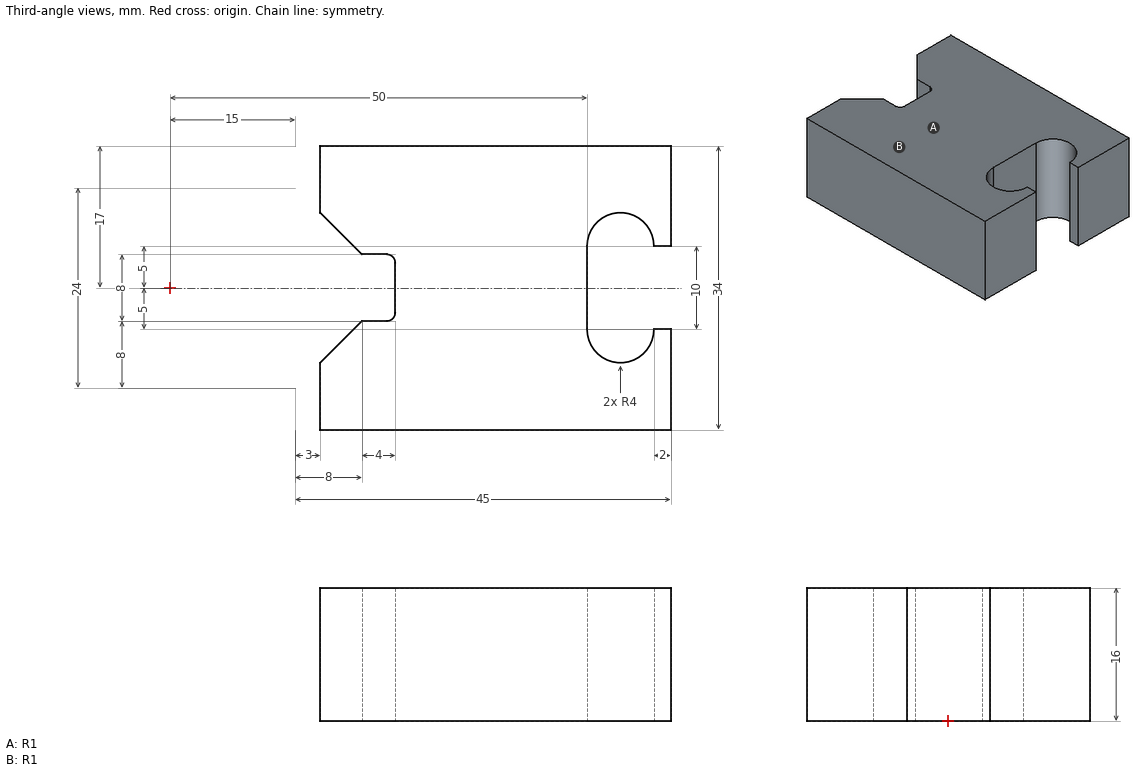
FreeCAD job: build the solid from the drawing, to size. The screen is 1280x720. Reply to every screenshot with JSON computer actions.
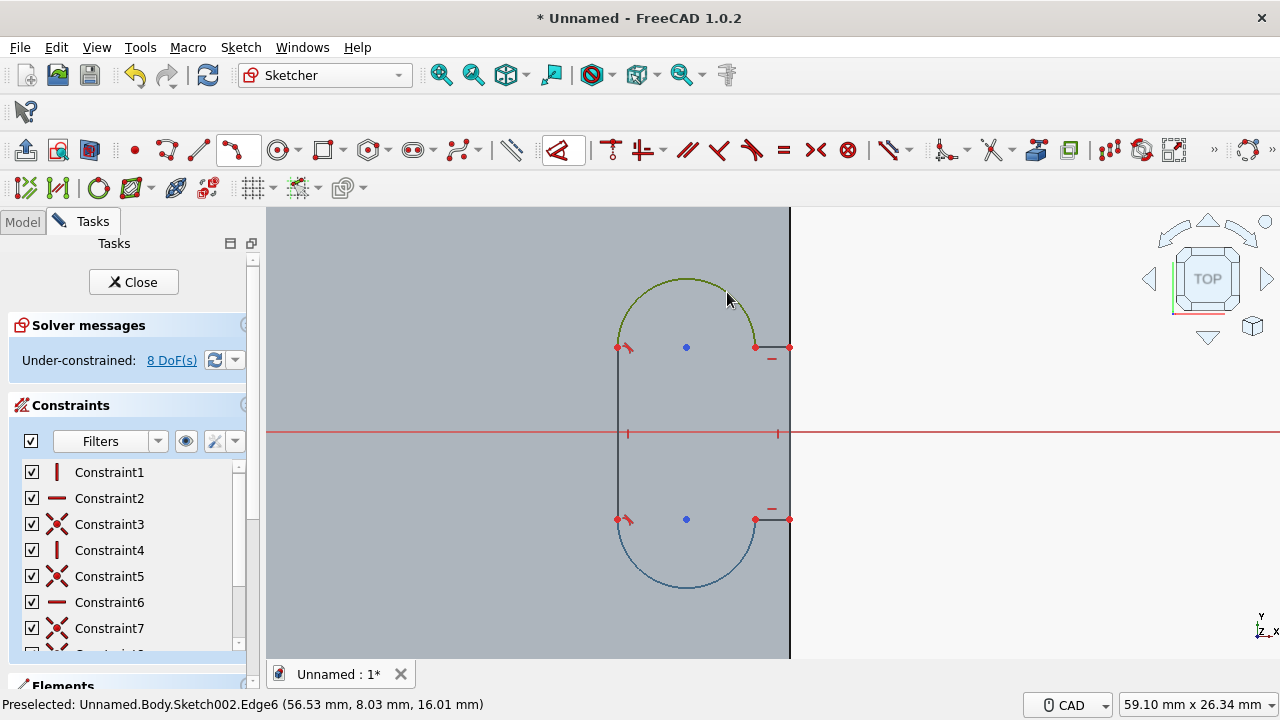
{"action": "left_click", "coordinate": [784, 150]}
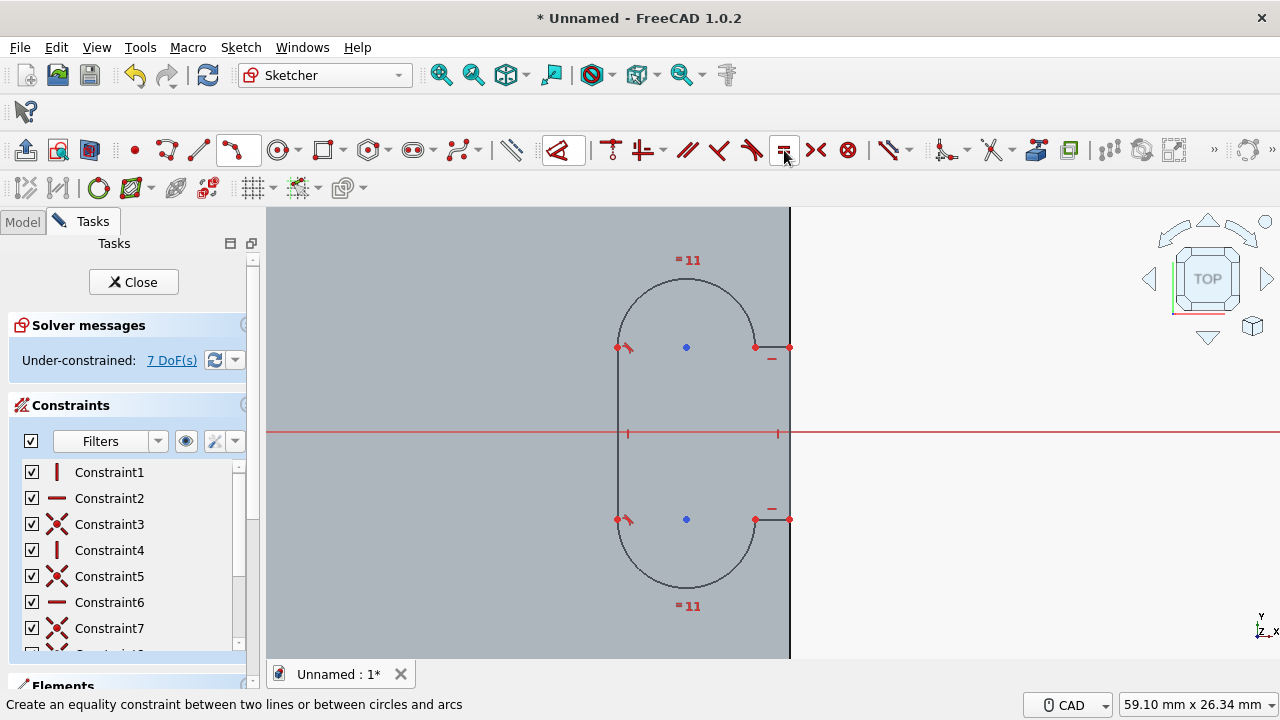
{"action": "left_click", "coordinate": [646, 575]}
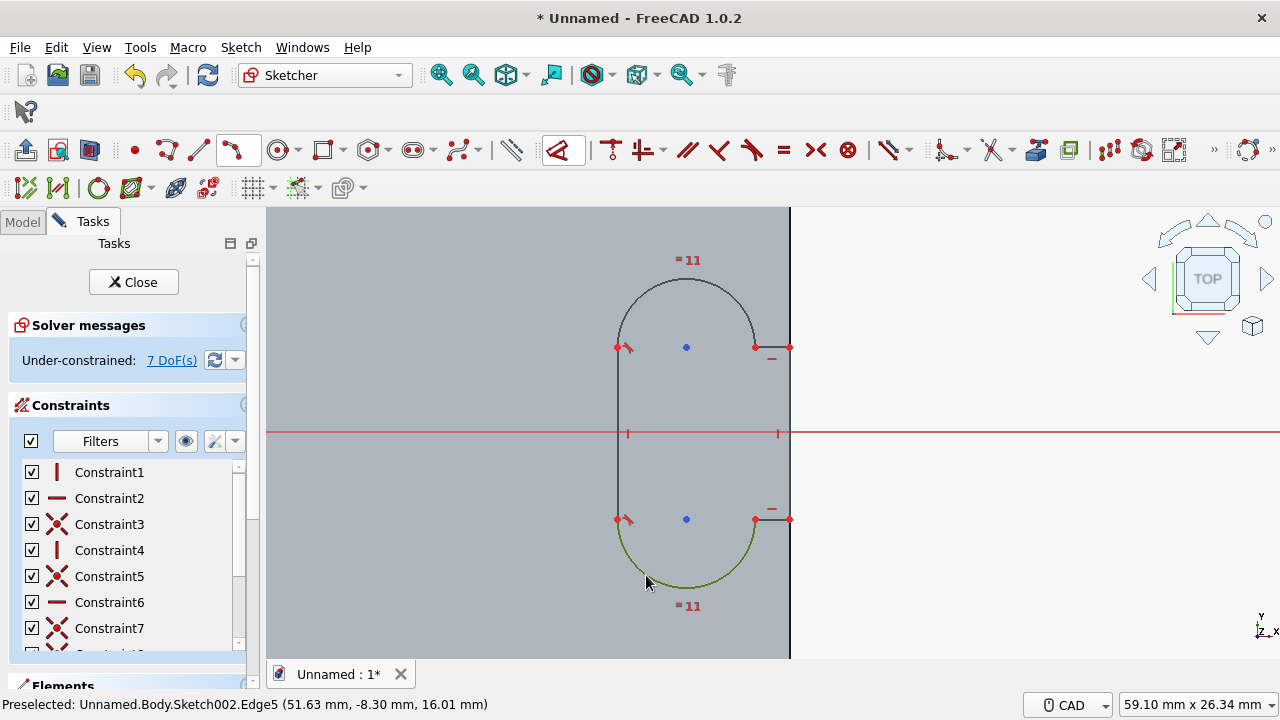
{"action": "left_click", "coordinate": [580, 150]}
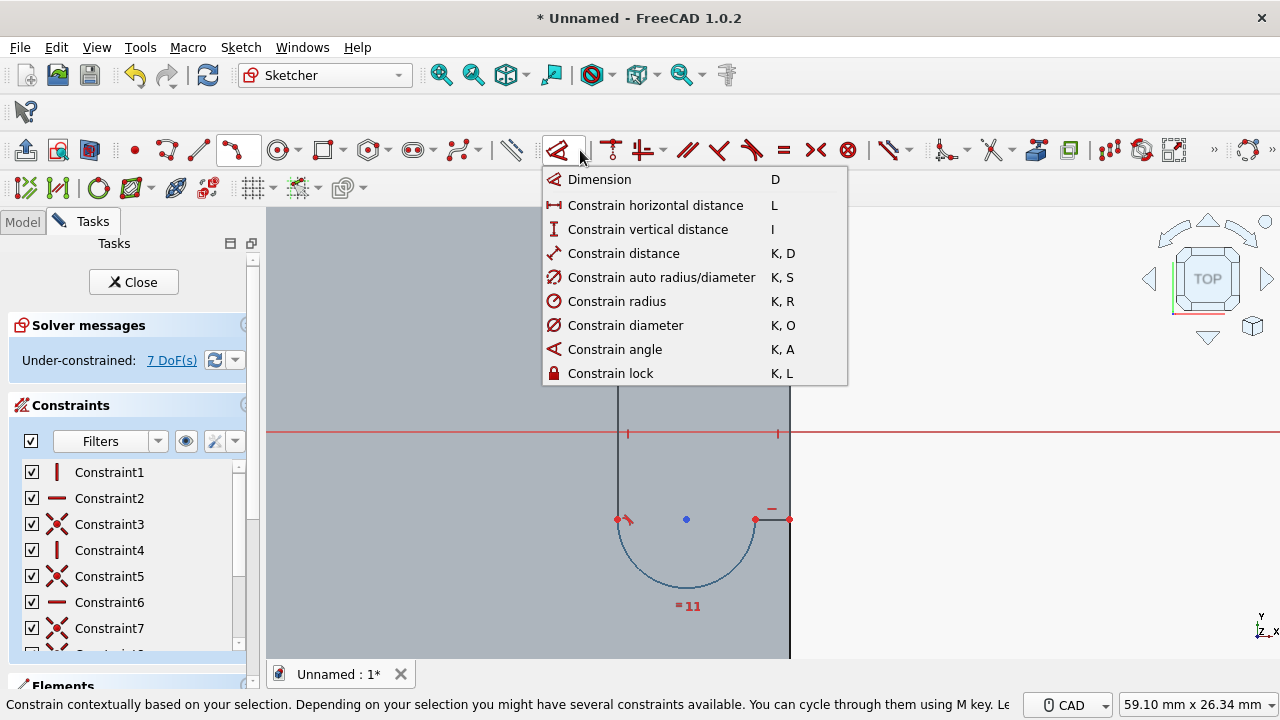
{"action": "left_click", "coordinate": [695, 301]}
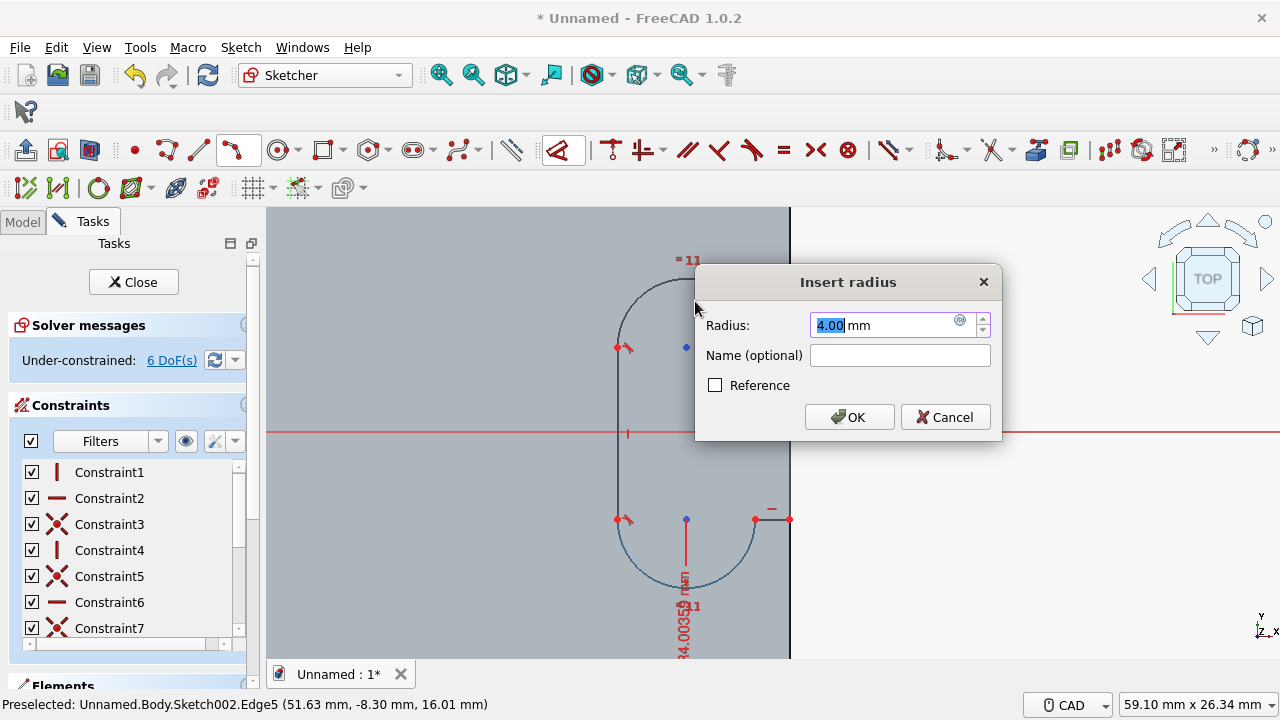
{"action": "type", "text": "4"}
{"action": "key", "text": "Return"}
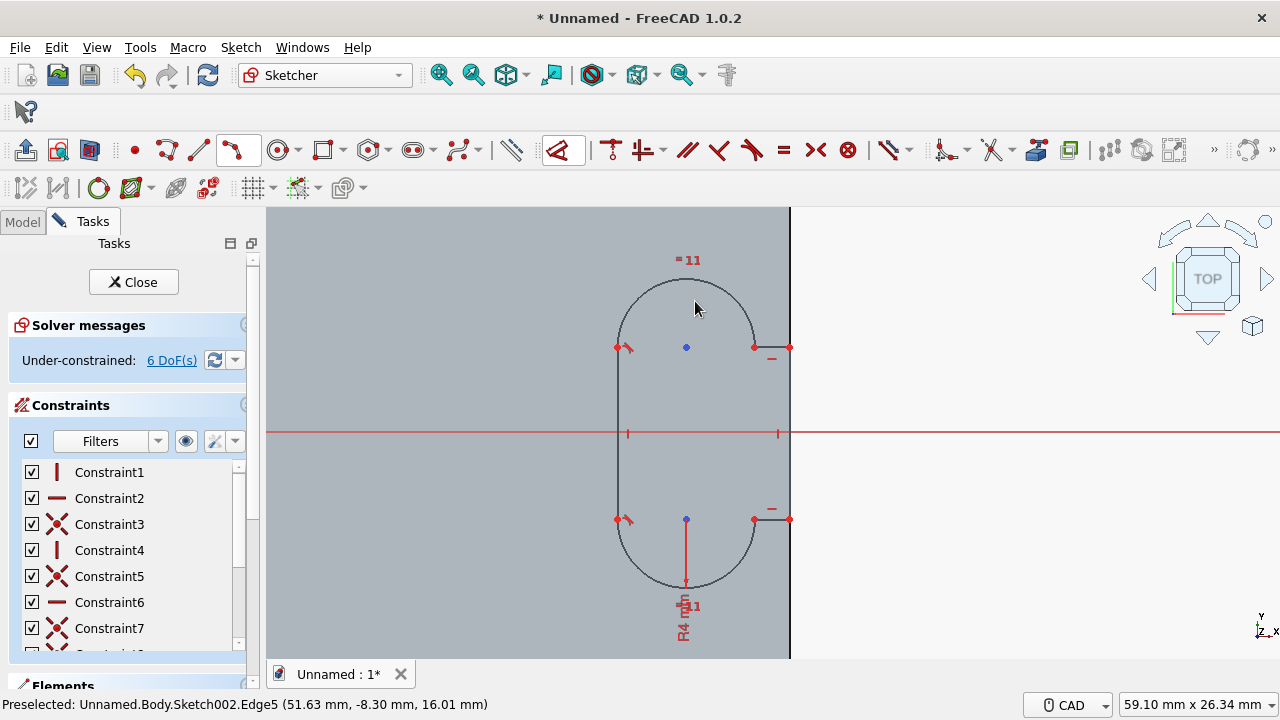
{"action": "scroll", "coordinate": [765, 520], "scroll_direction": "up", "scroll_amount": 2}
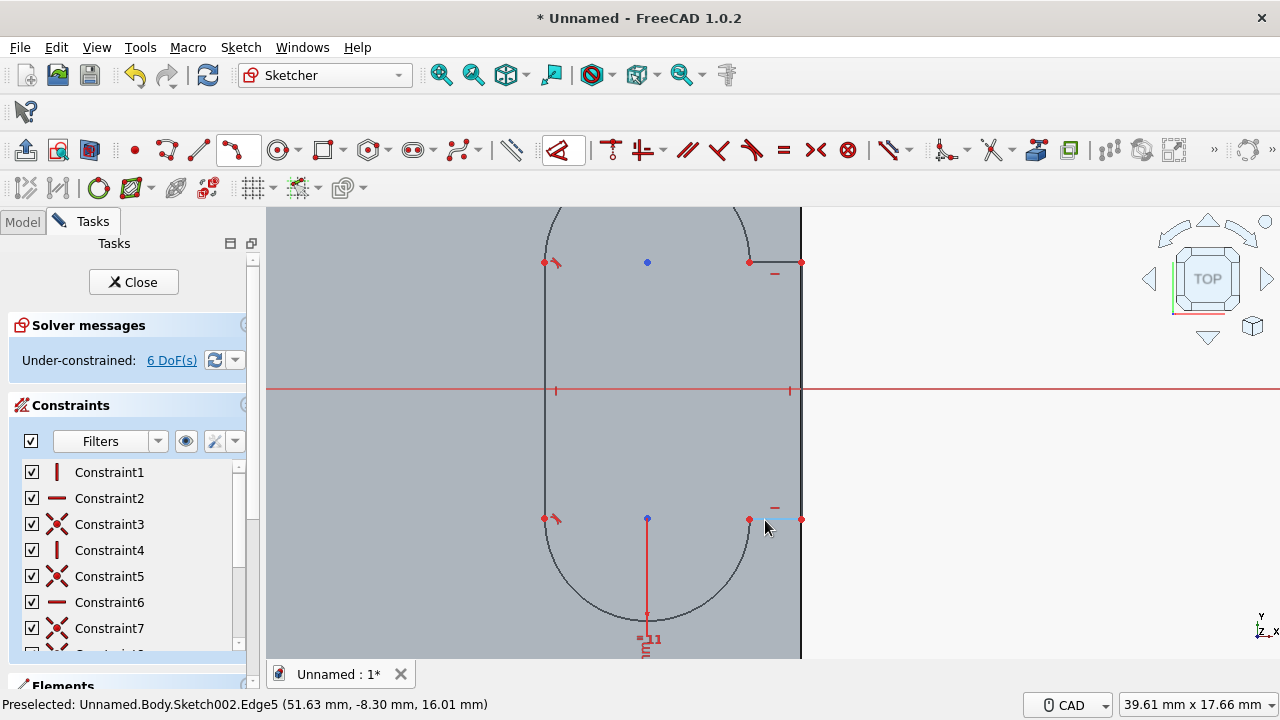
{"action": "left_click", "coordinate": [765, 519]}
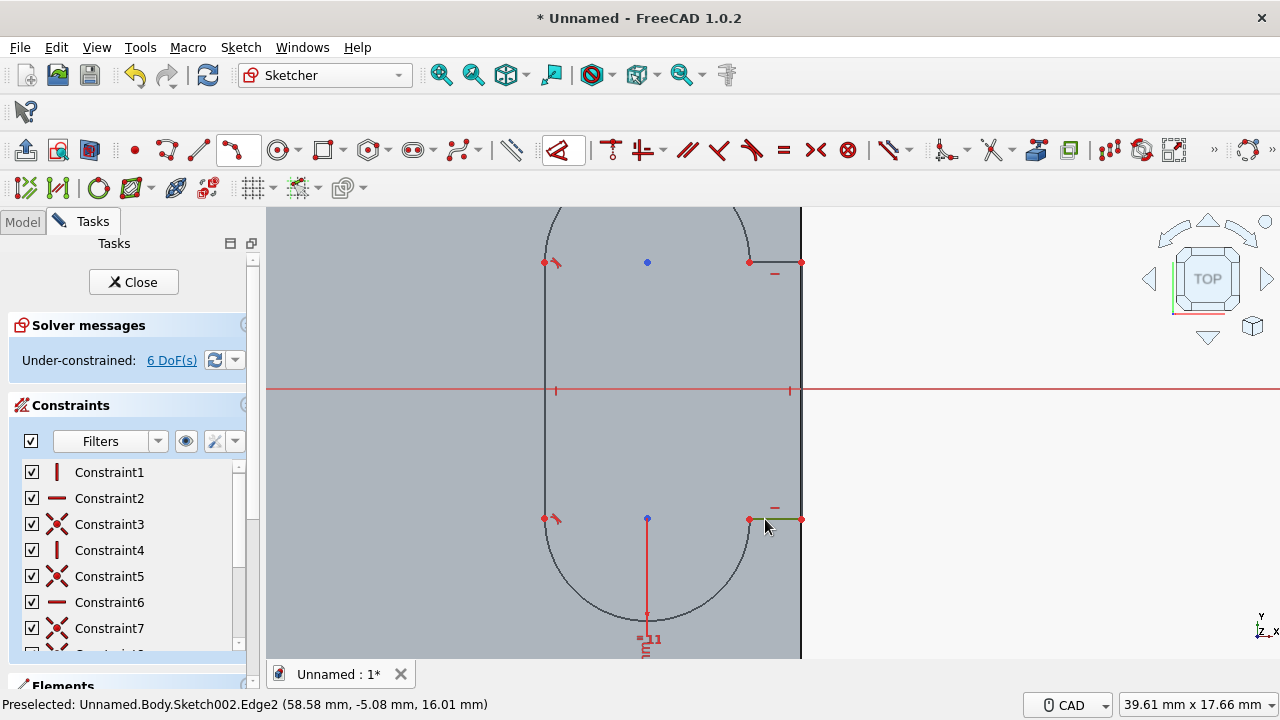
{"action": "key", "text": "l"}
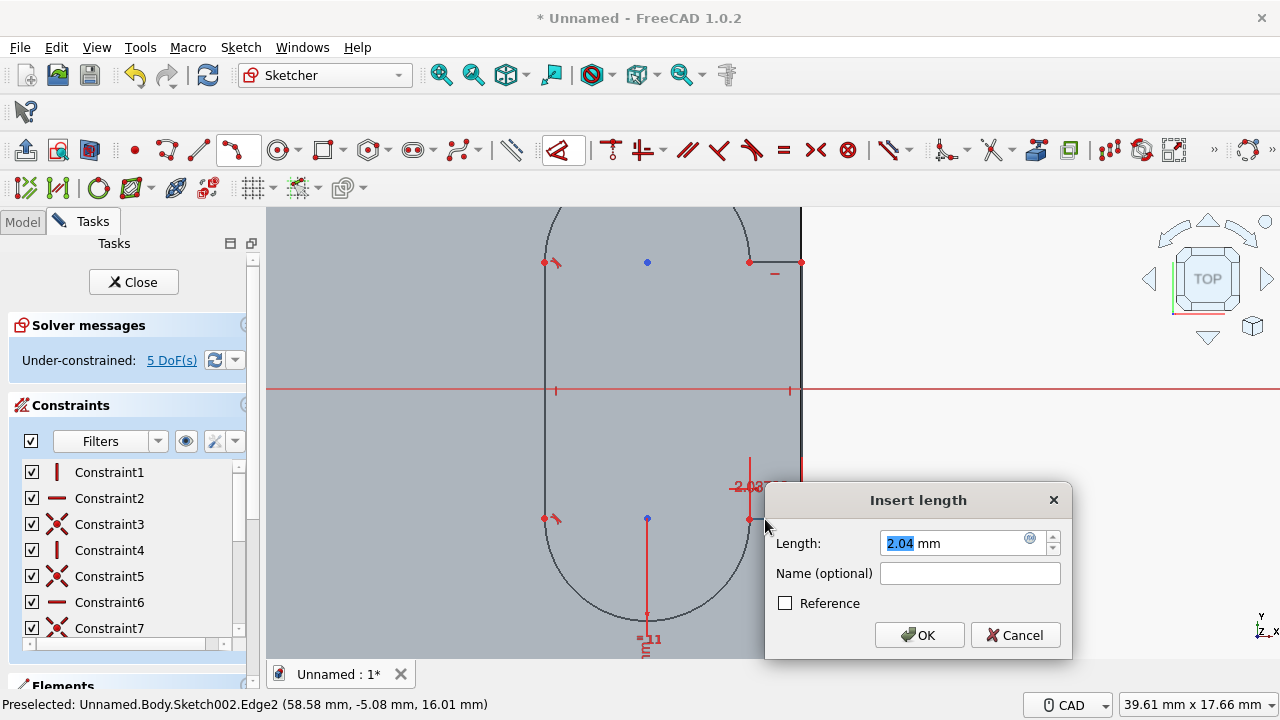
{"action": "type", "text": "2"}
{"action": "key", "text": "Return"}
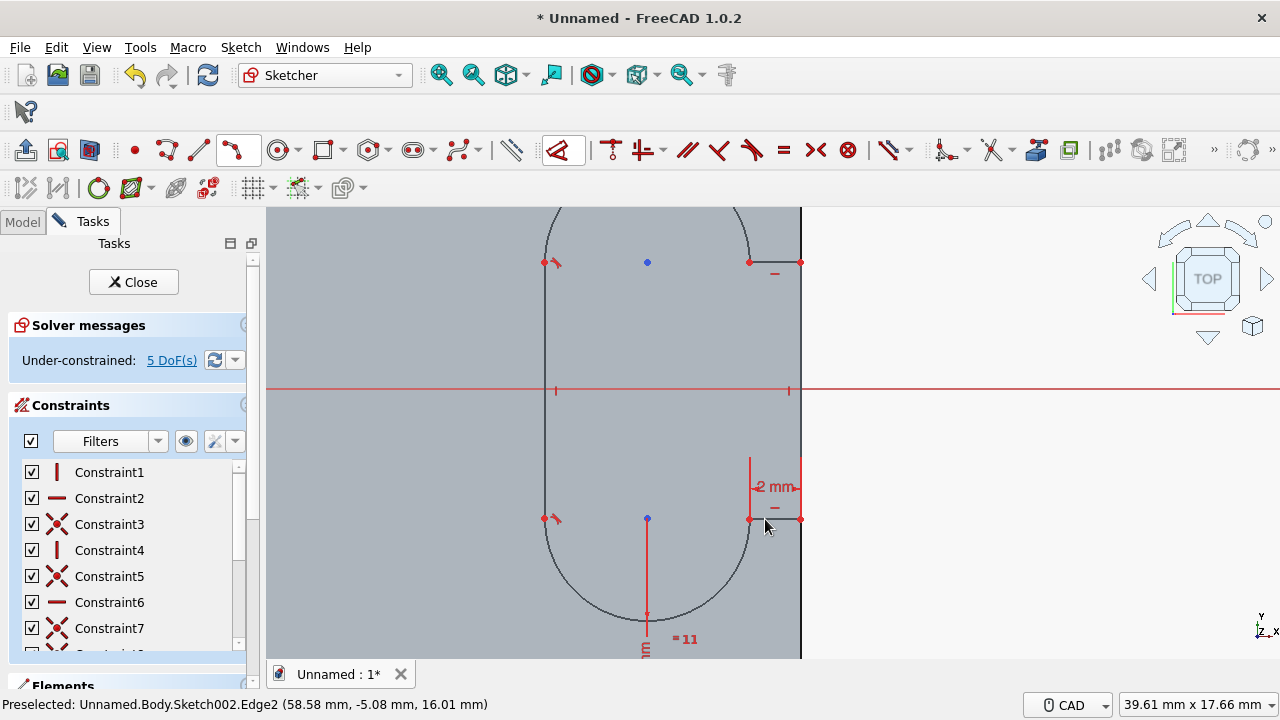
{"action": "left_click", "coordinate": [545, 339]}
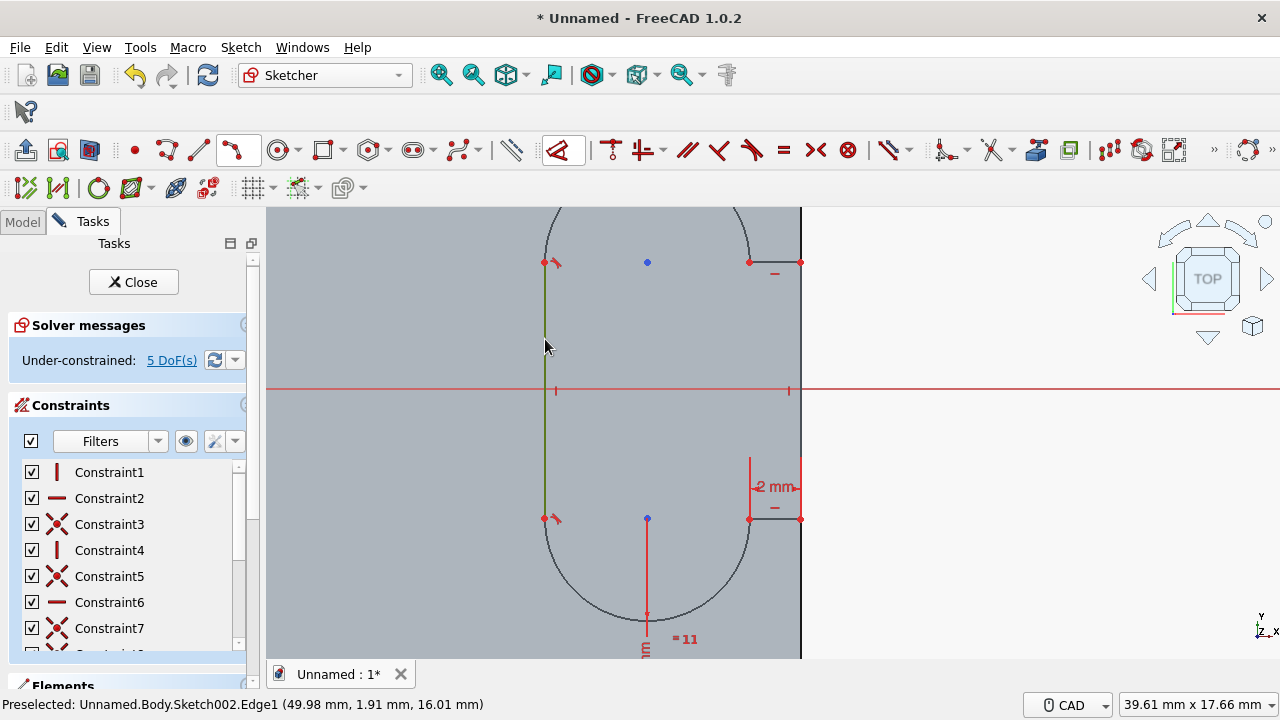
{"action": "left_click", "coordinate": [580, 150]}